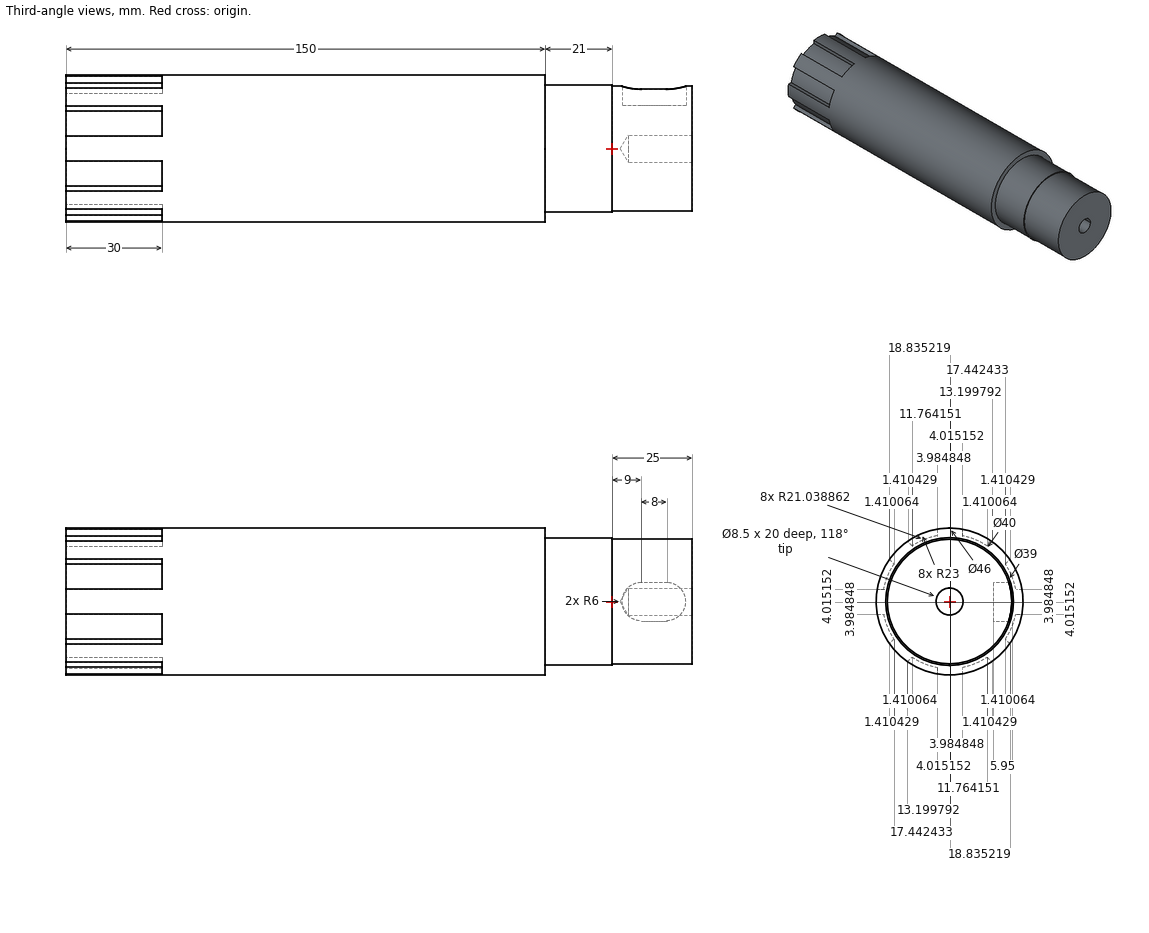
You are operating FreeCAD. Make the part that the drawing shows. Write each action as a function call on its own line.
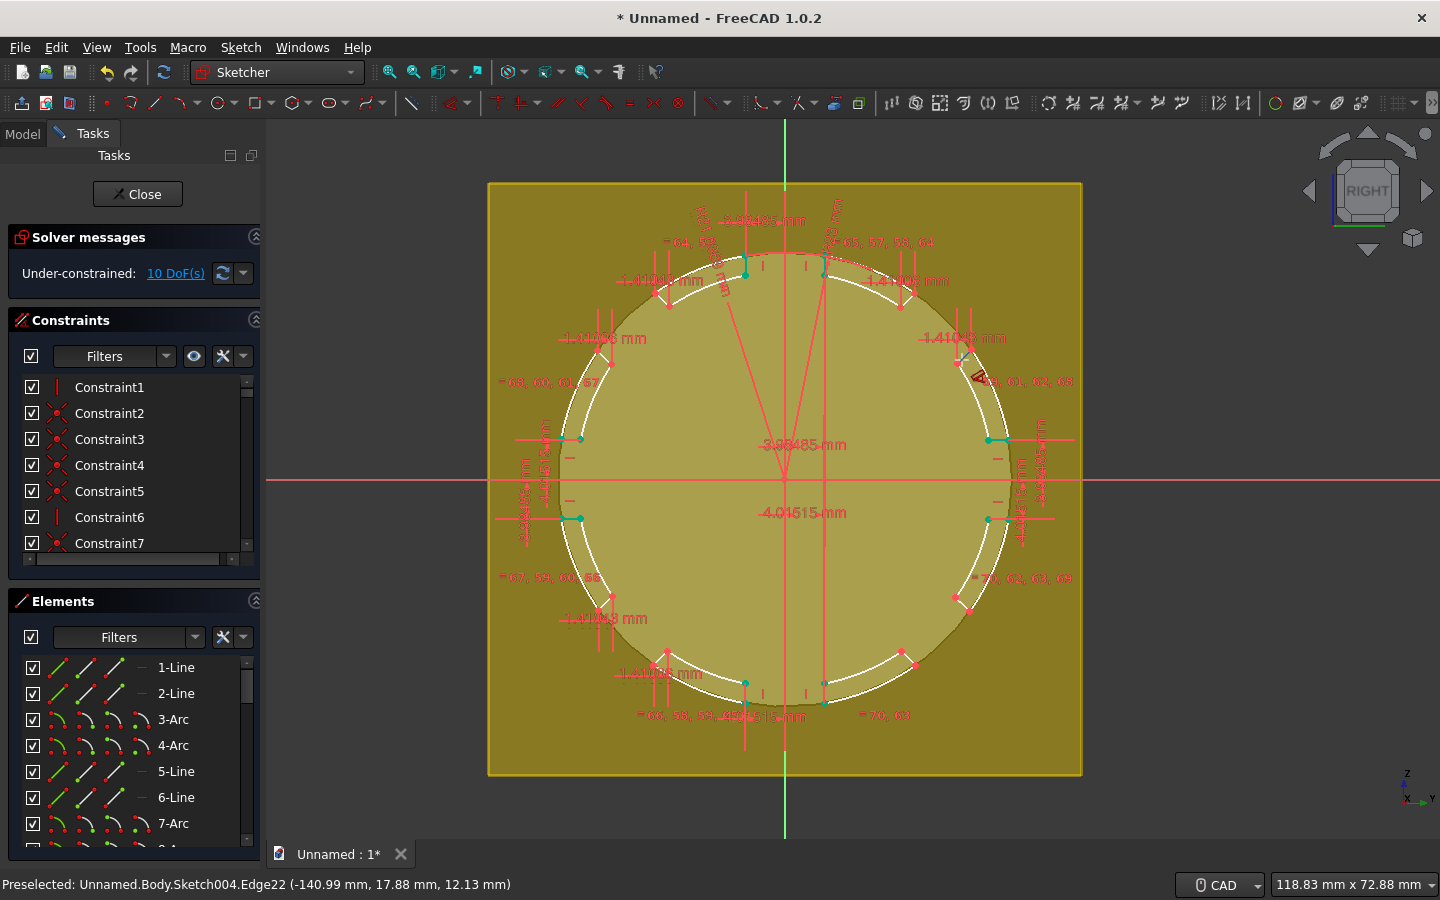
scroll(966, 607, up, 6)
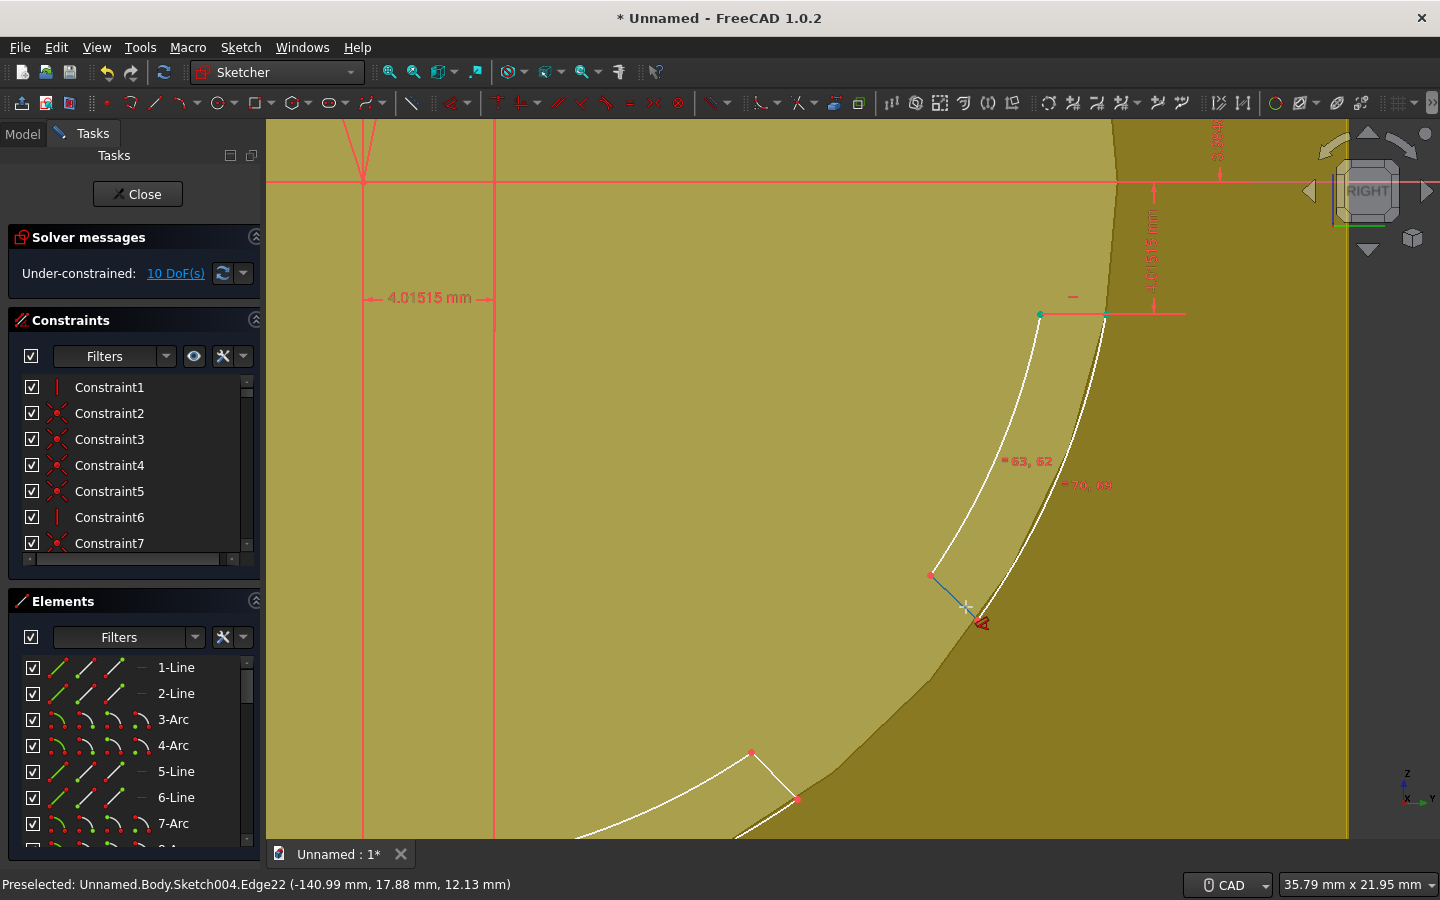
click(964, 607)
click(954, 654)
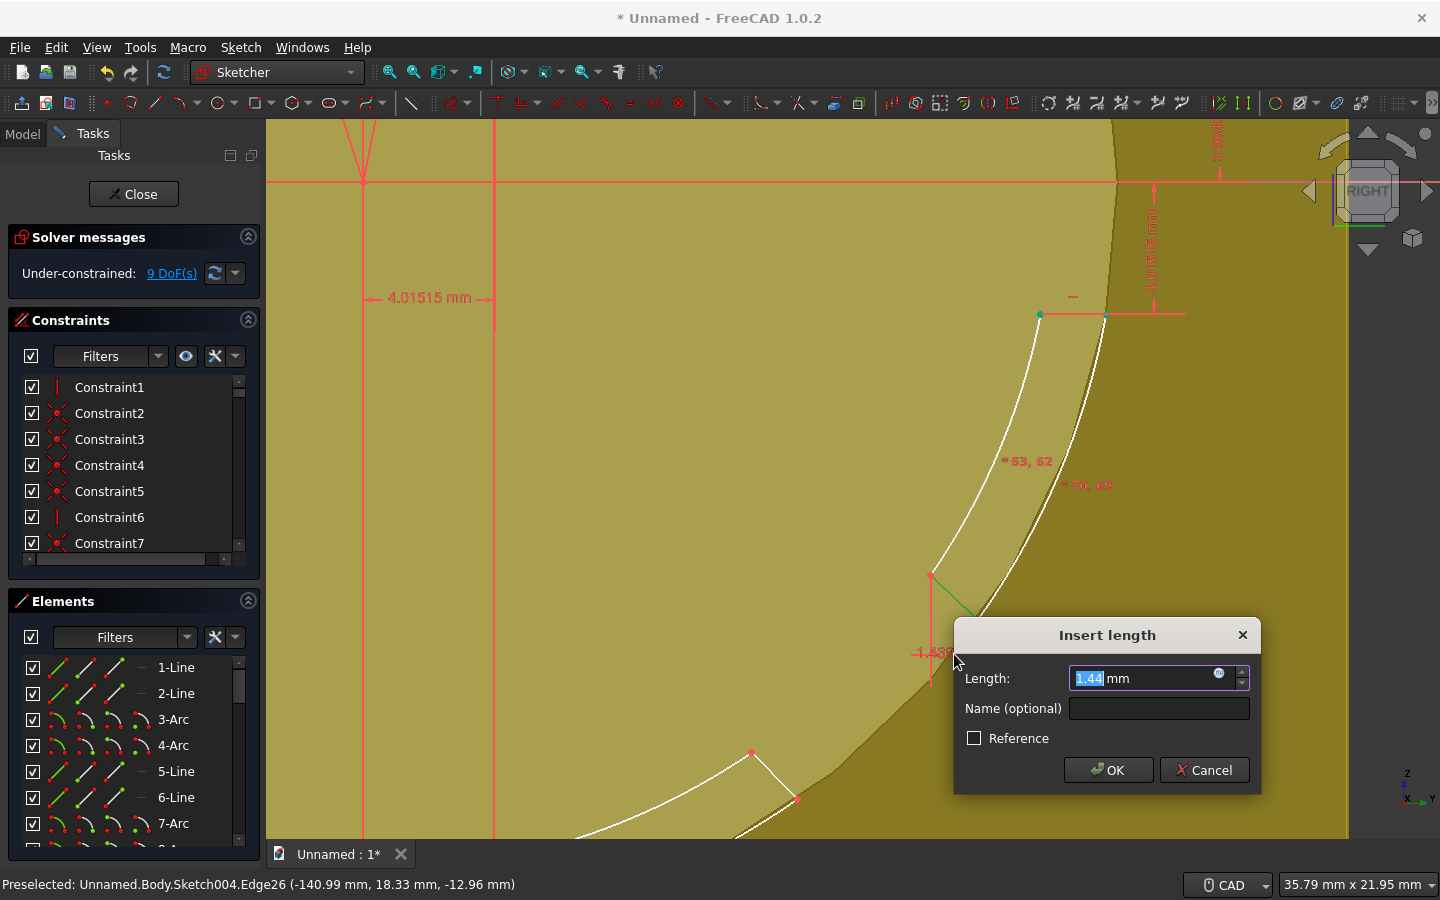
text(1.410064)
key(Return)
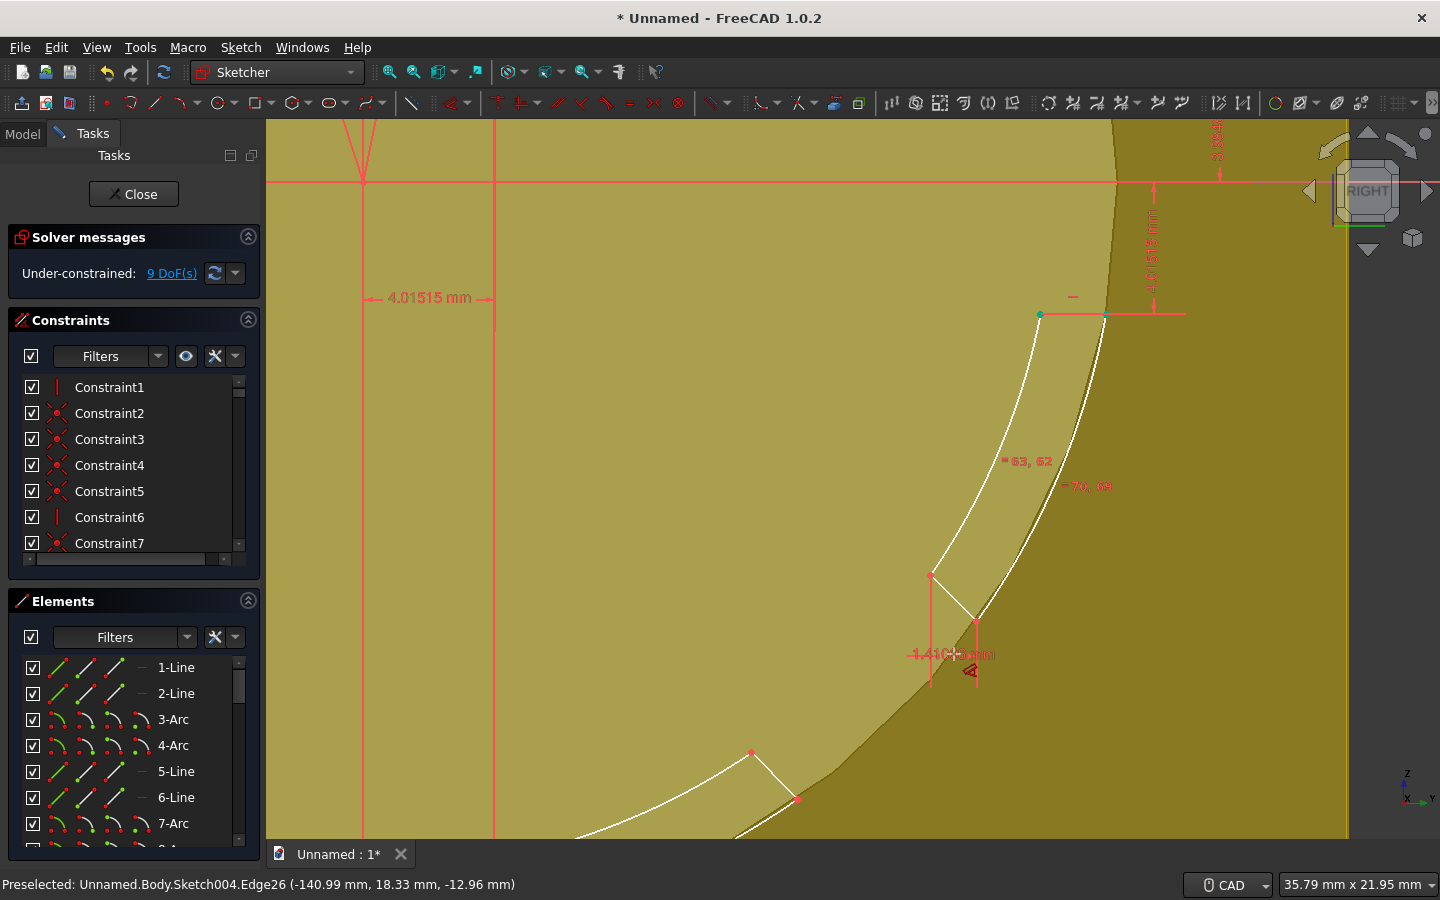
click(766, 767)
click(775, 719)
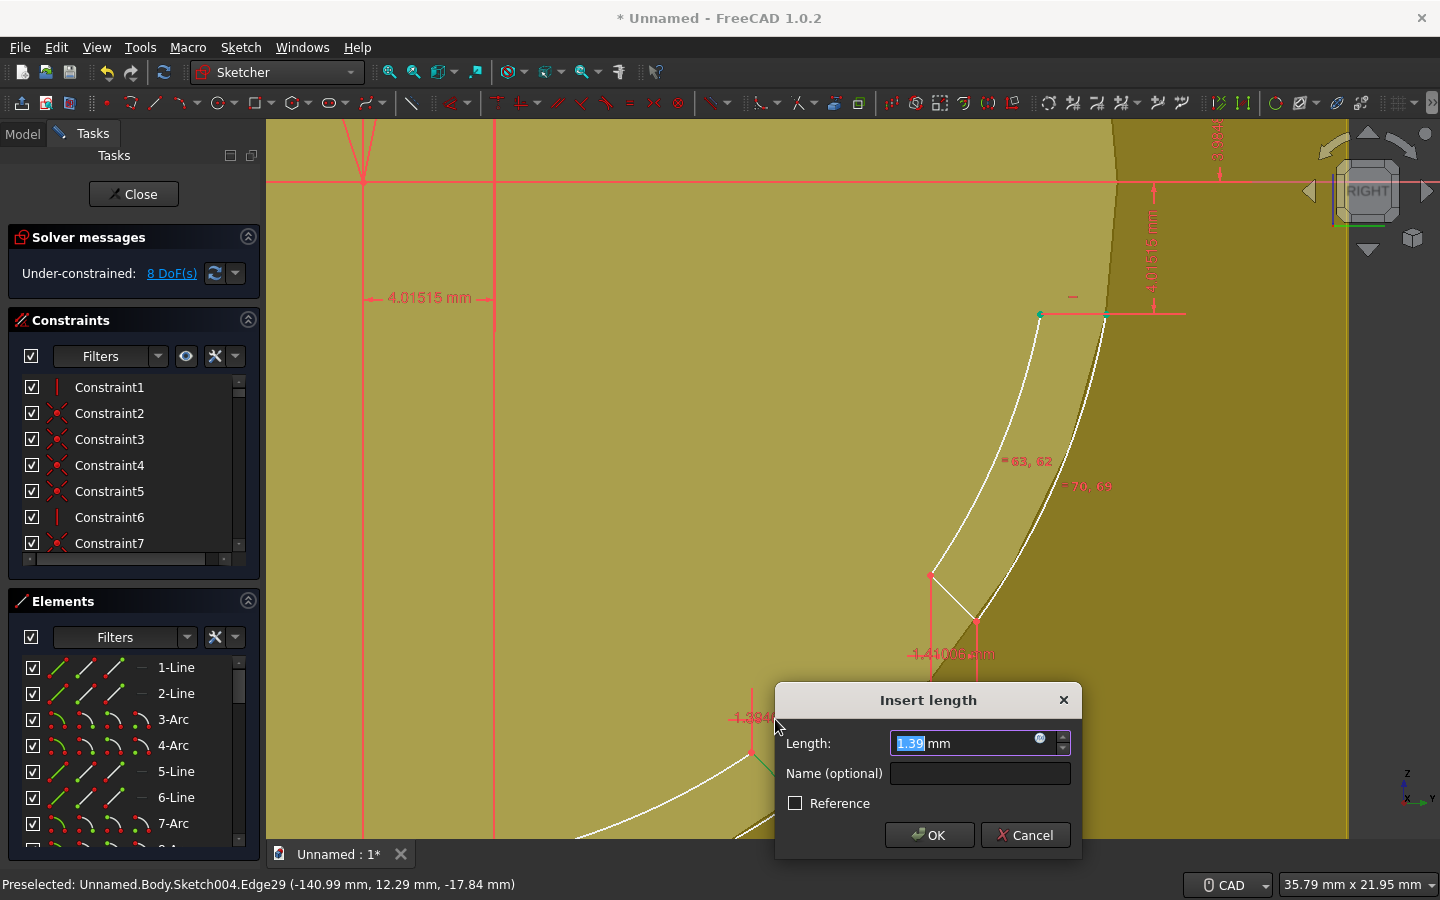
text(1.410429)
key(Return)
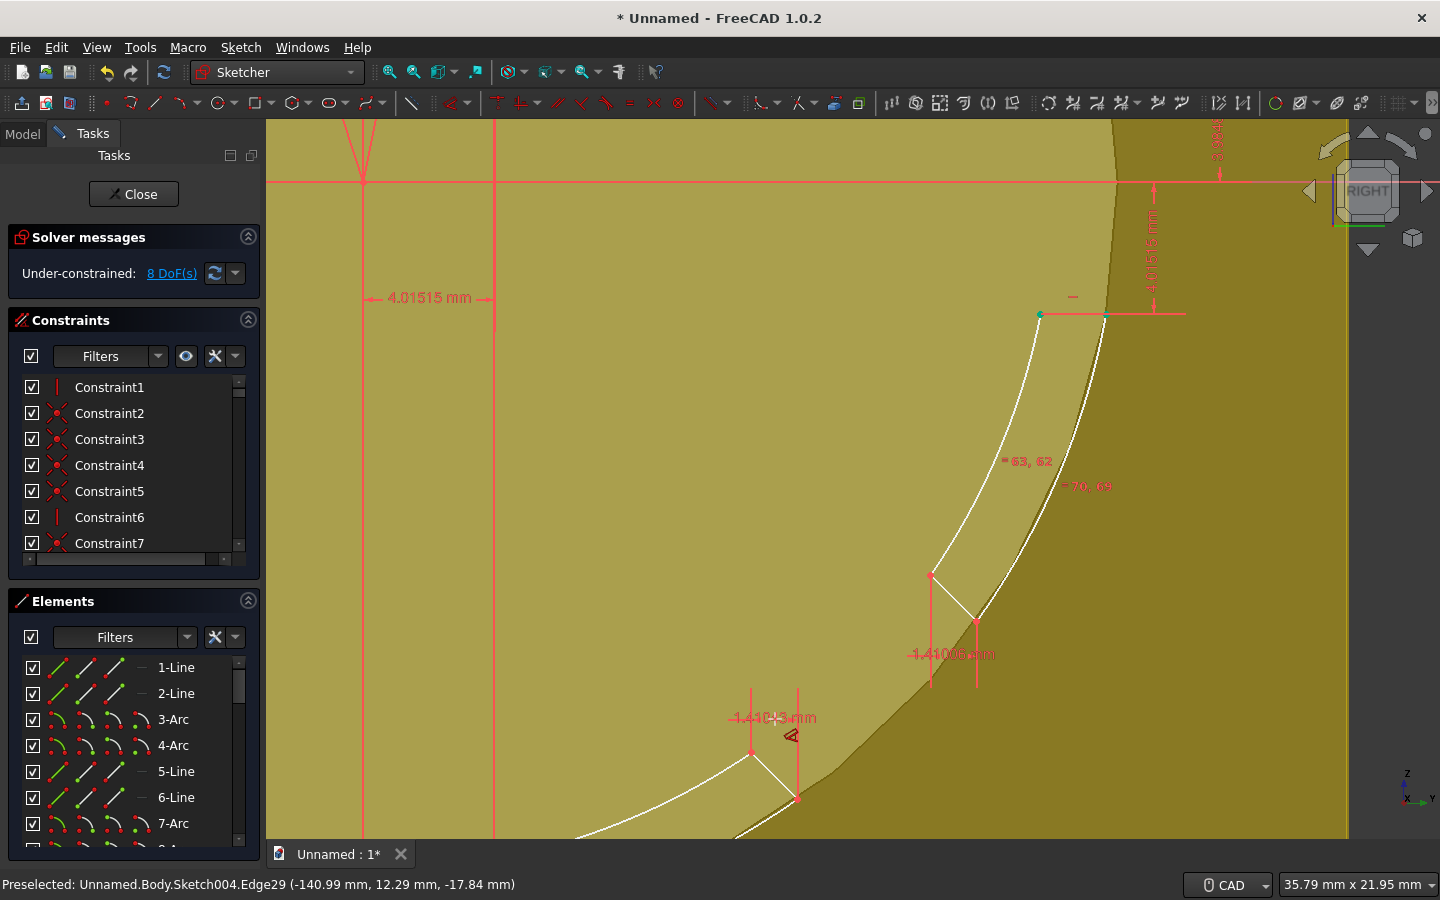
scroll(966, 607, down, 6)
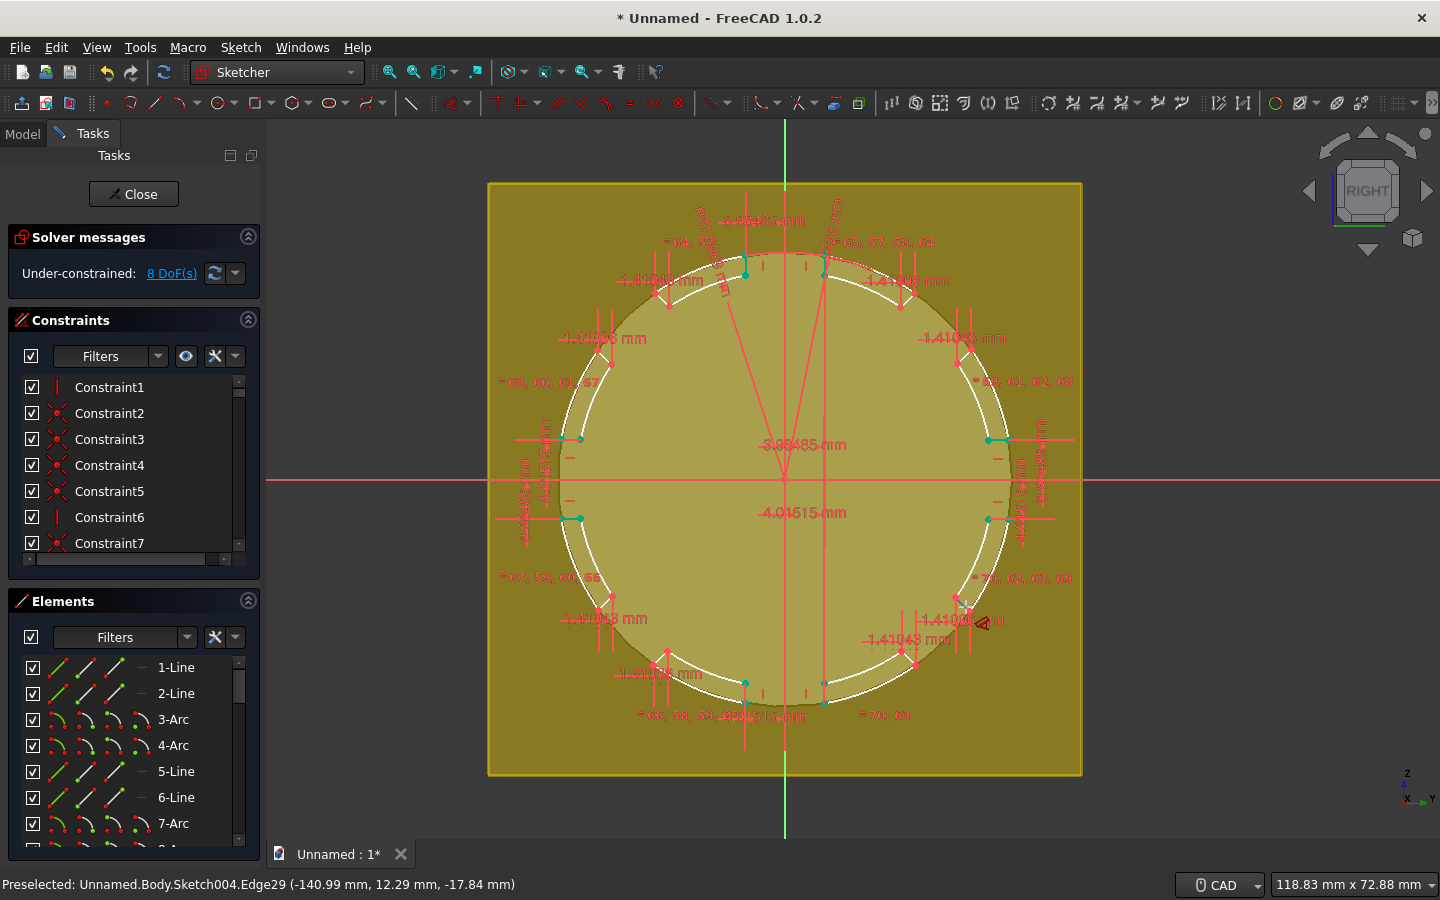
click(669, 307)
click(768, 273)